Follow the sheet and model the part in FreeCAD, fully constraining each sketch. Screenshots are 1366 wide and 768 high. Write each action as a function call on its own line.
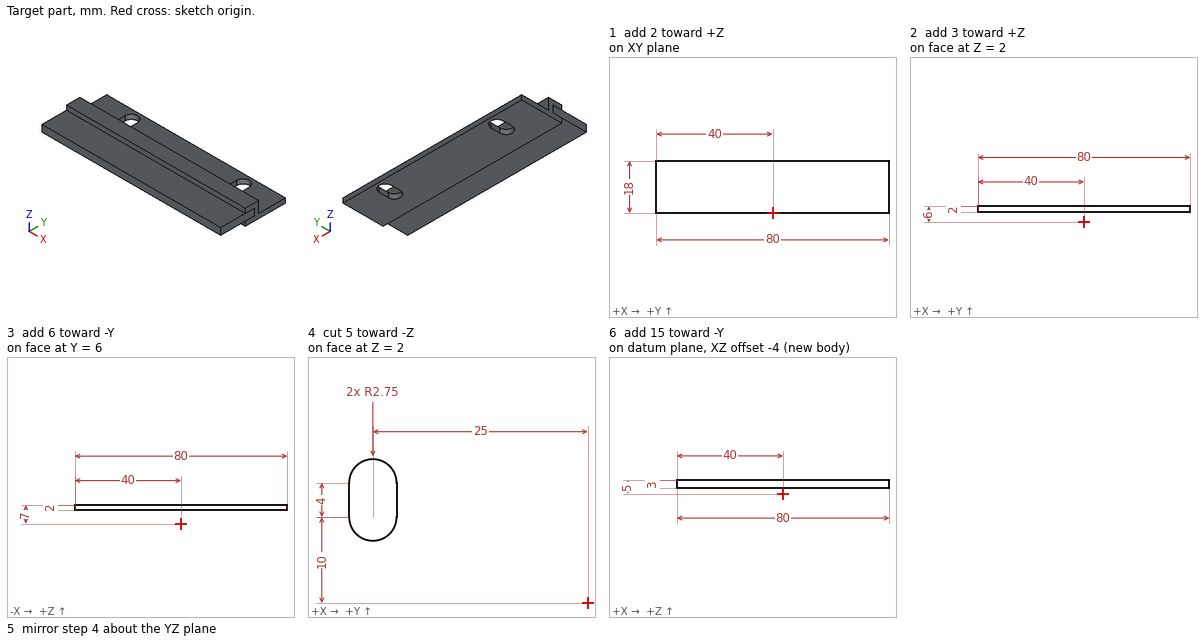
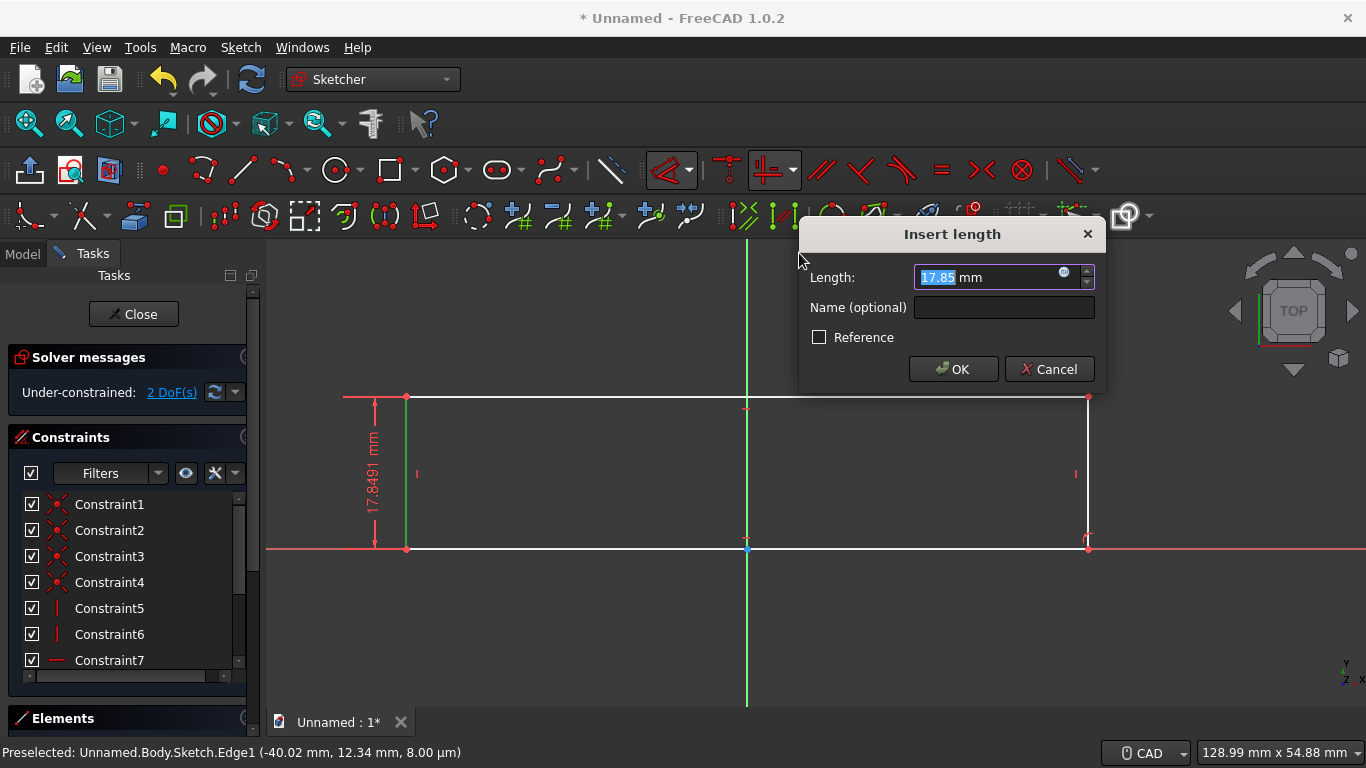
text(18)
key(Return)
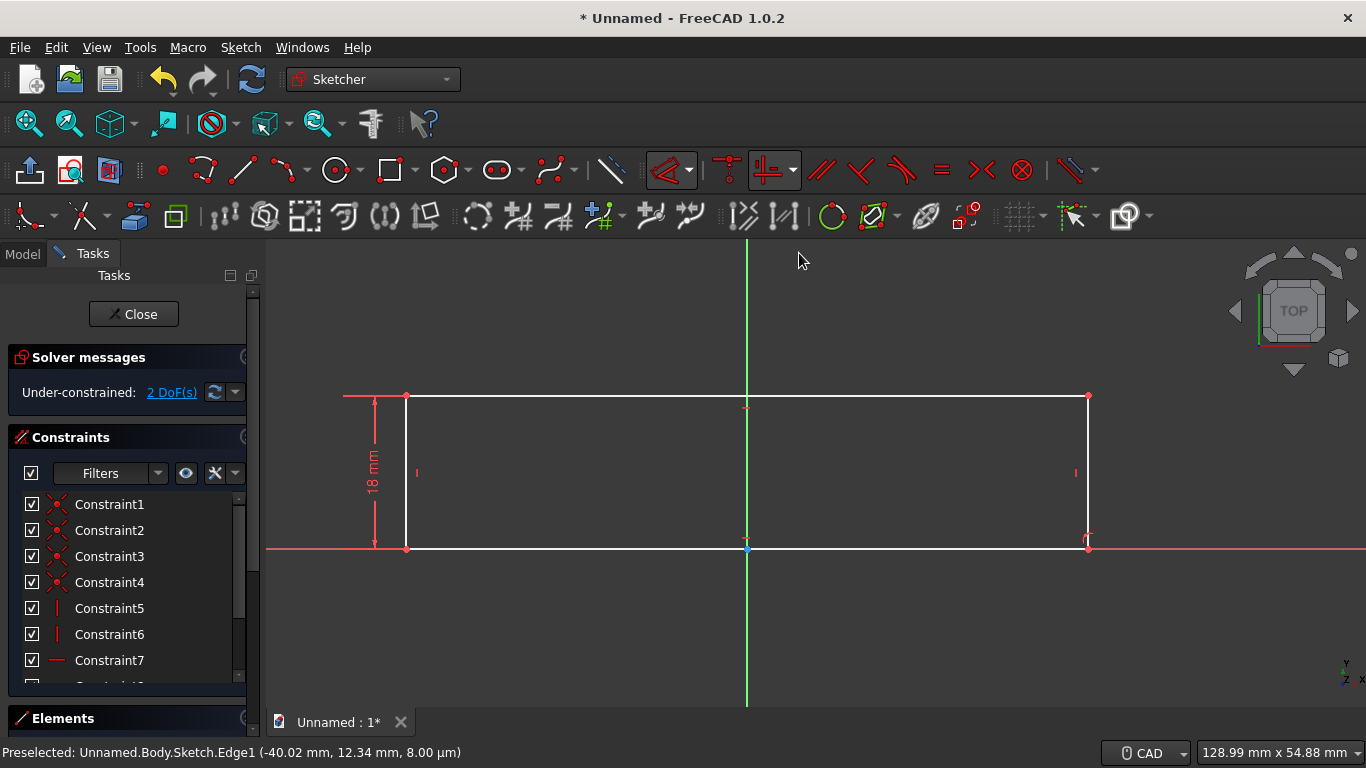
click(611, 549)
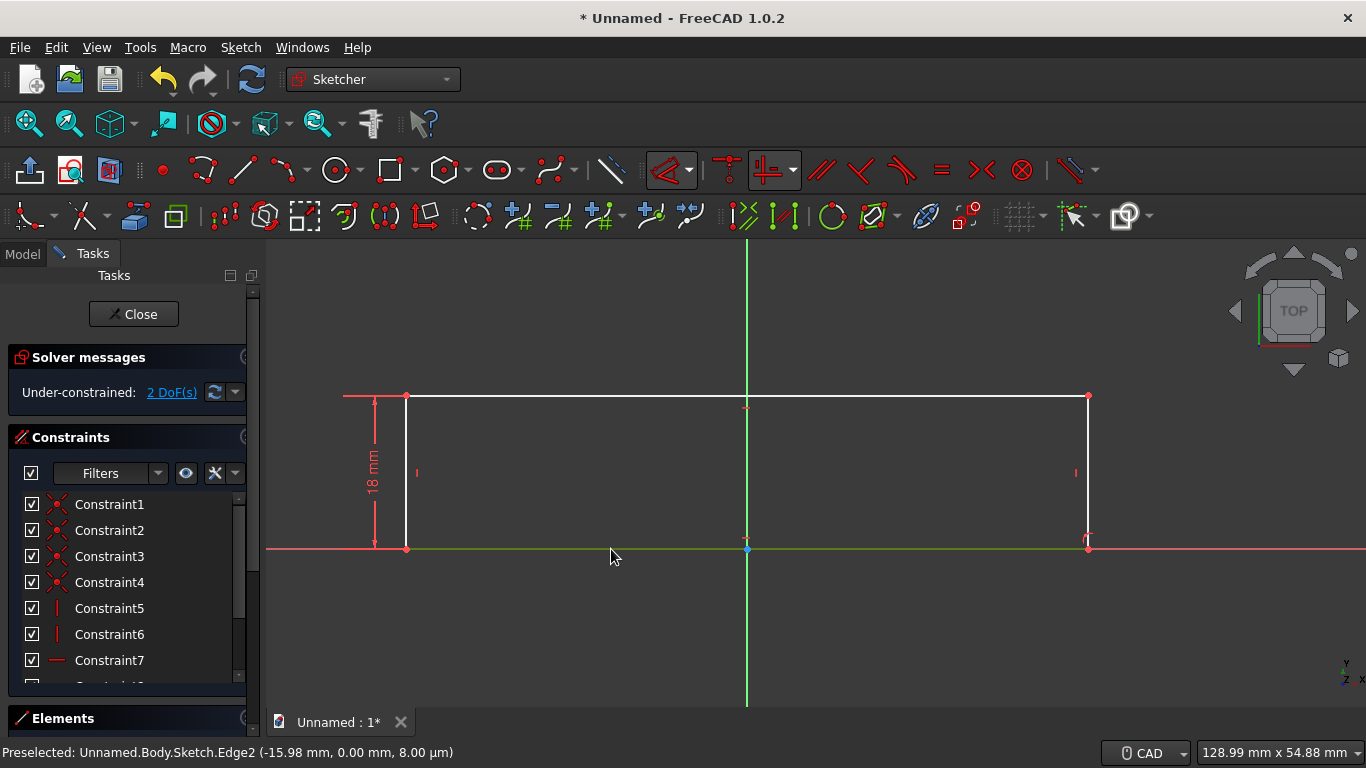
key(l)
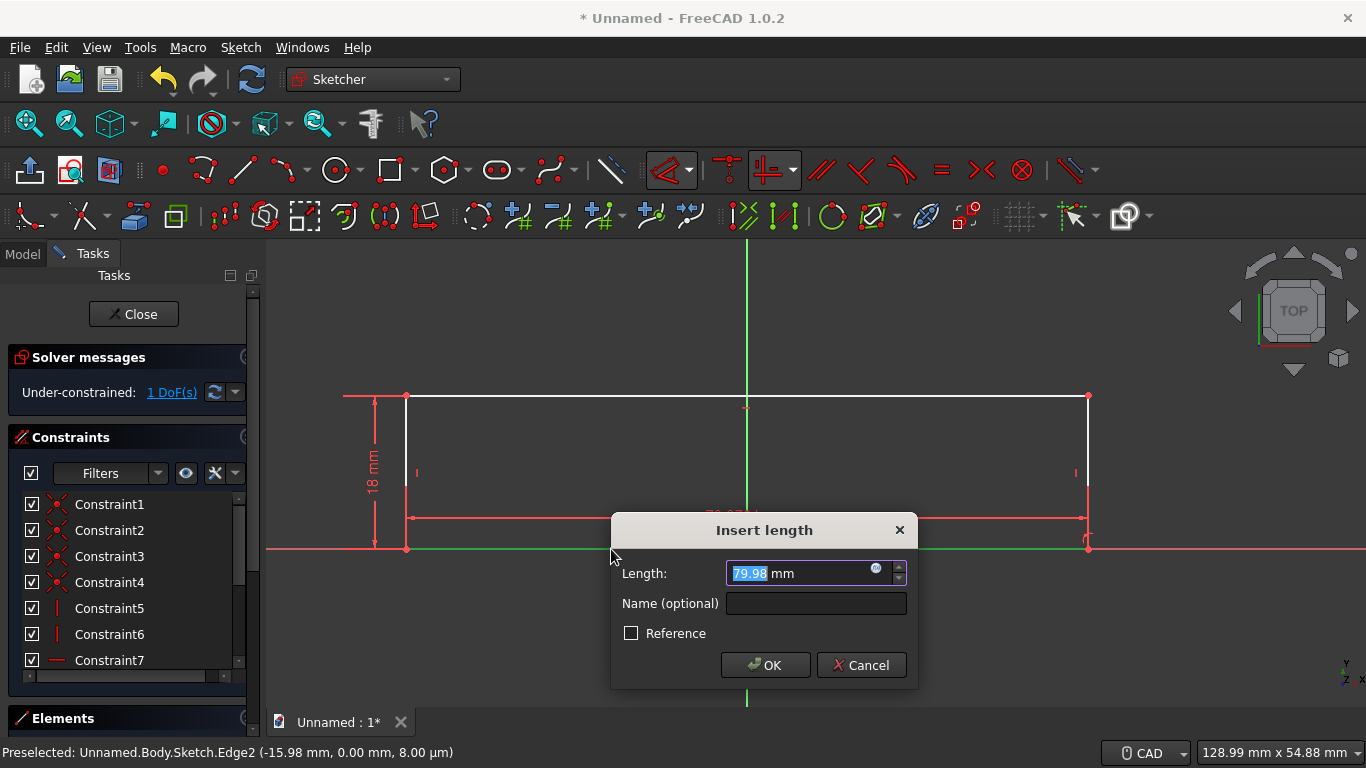
text(80)
key(Return)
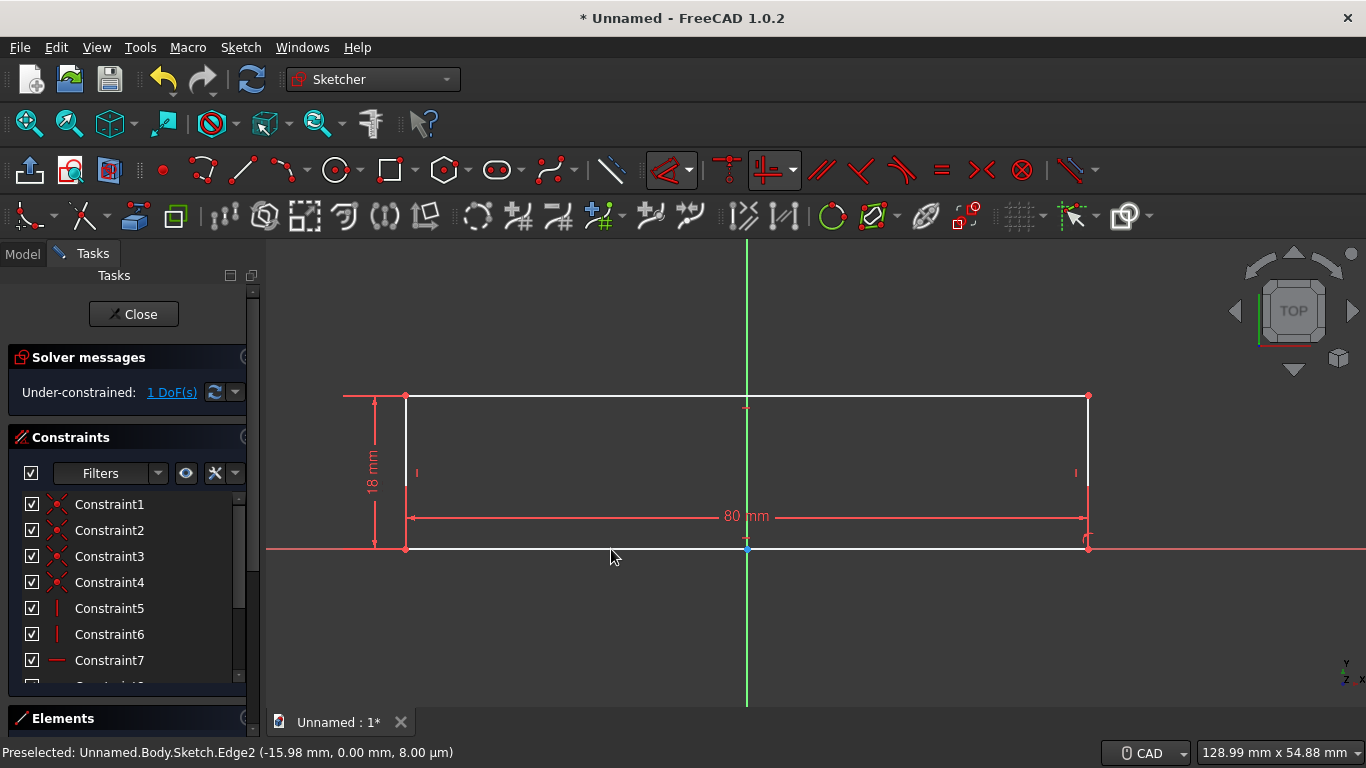
click(406, 396)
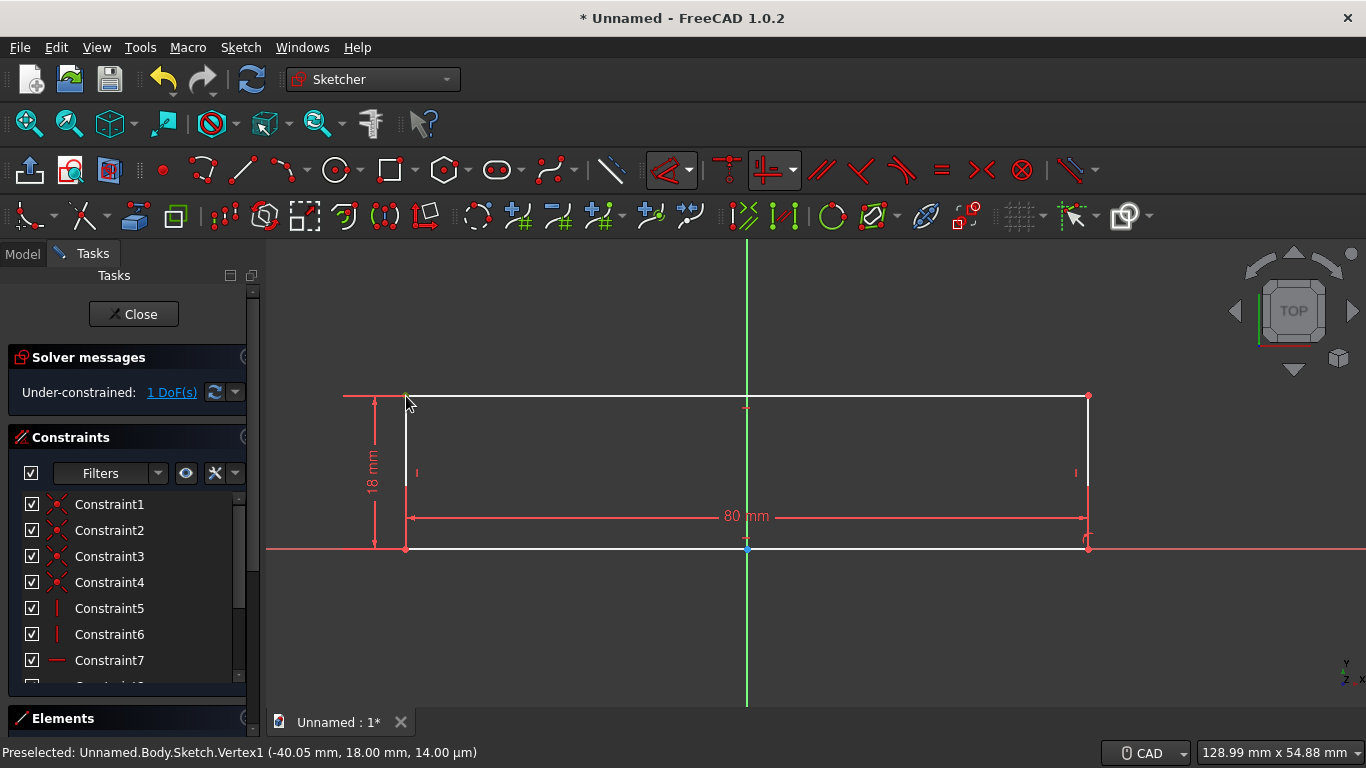
click(692, 170)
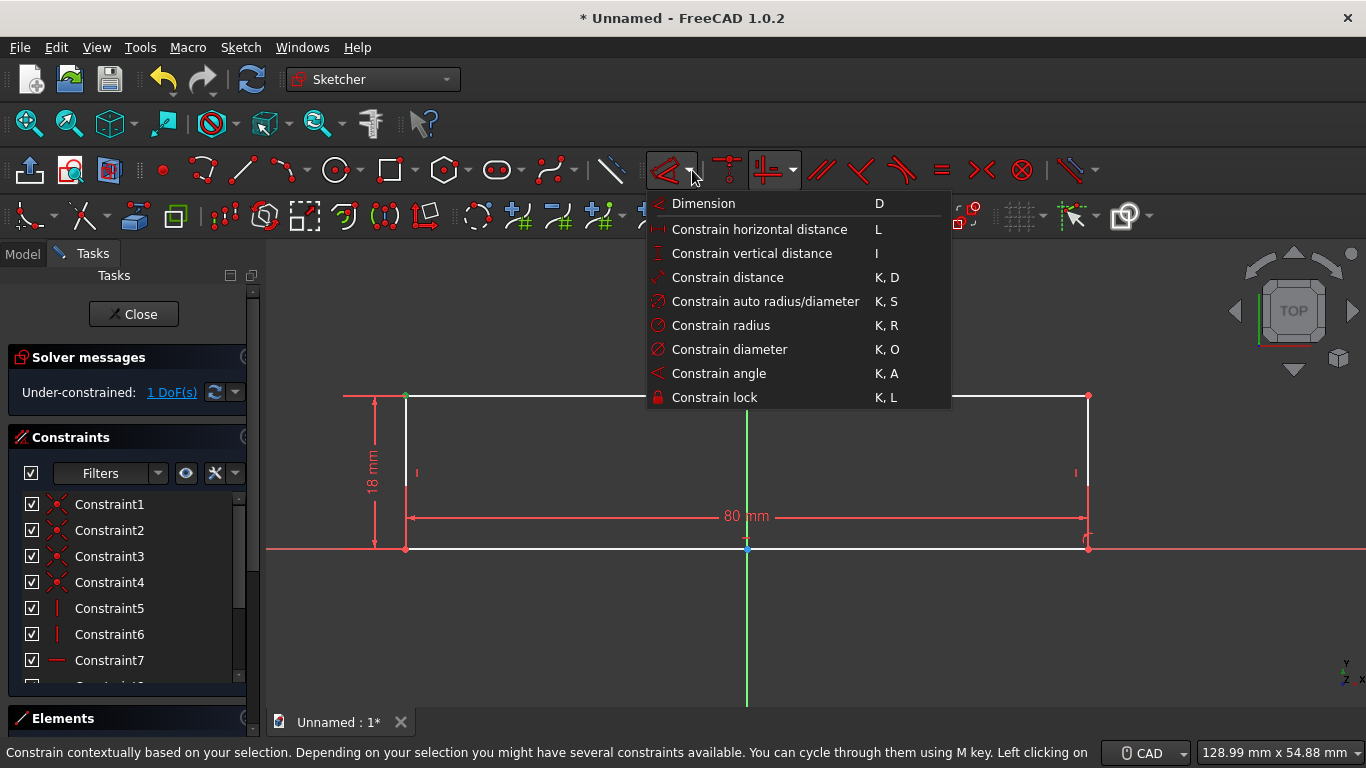
click(799, 229)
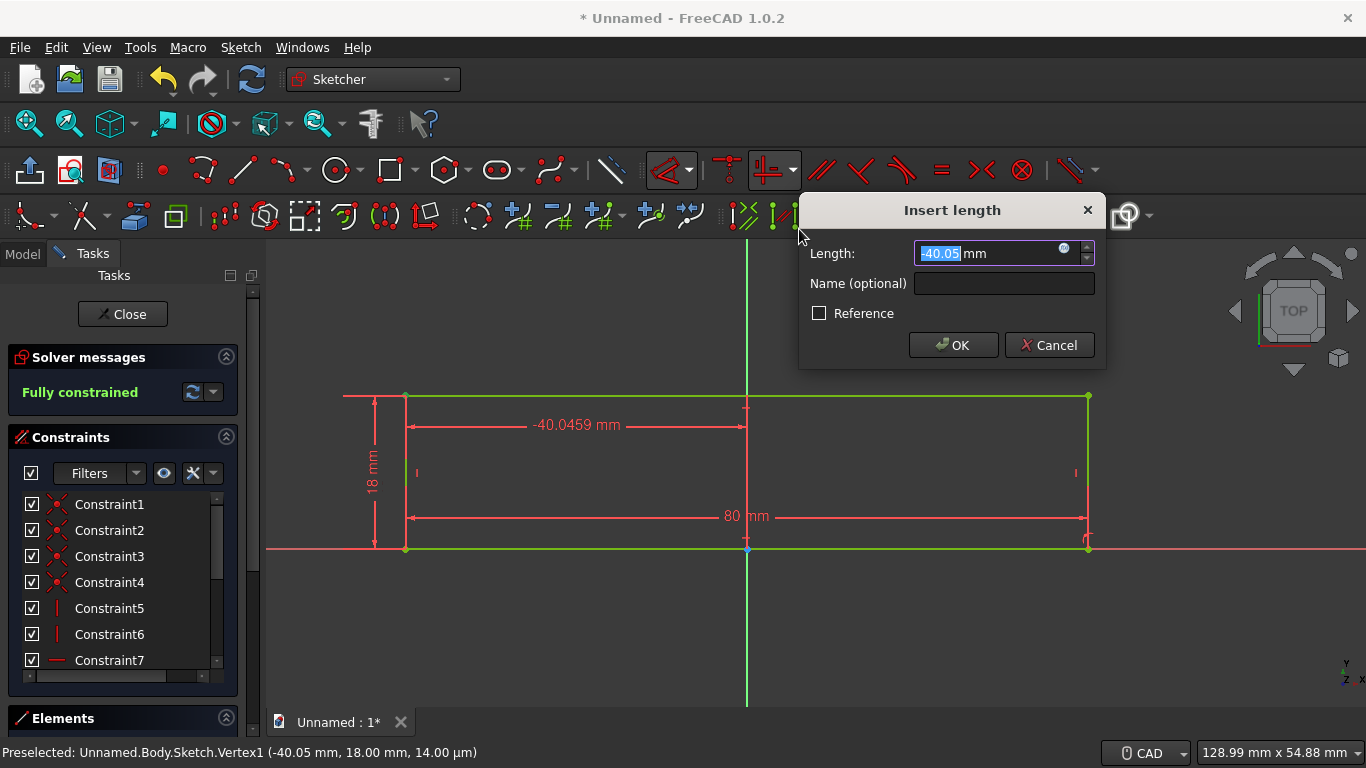
text(-40)
key(Return)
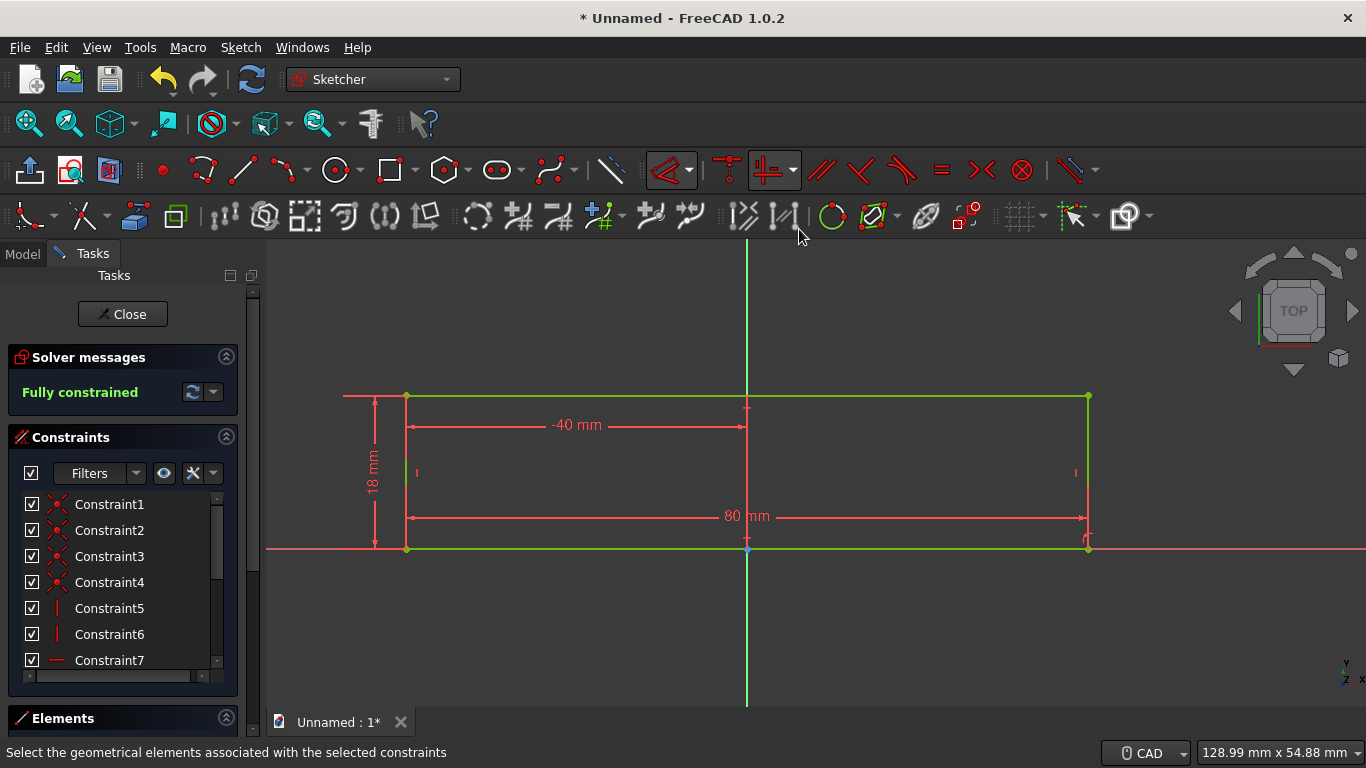
click(123, 314)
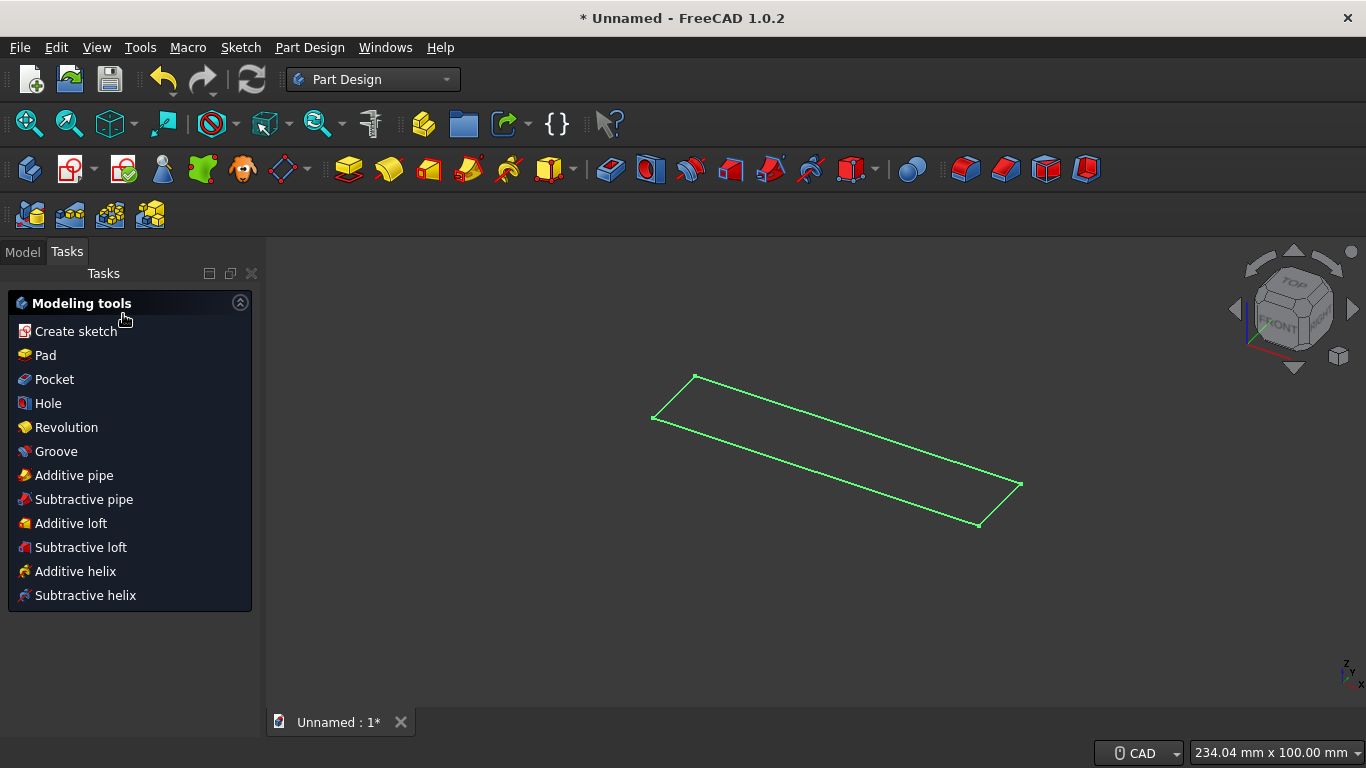
click(350, 170)